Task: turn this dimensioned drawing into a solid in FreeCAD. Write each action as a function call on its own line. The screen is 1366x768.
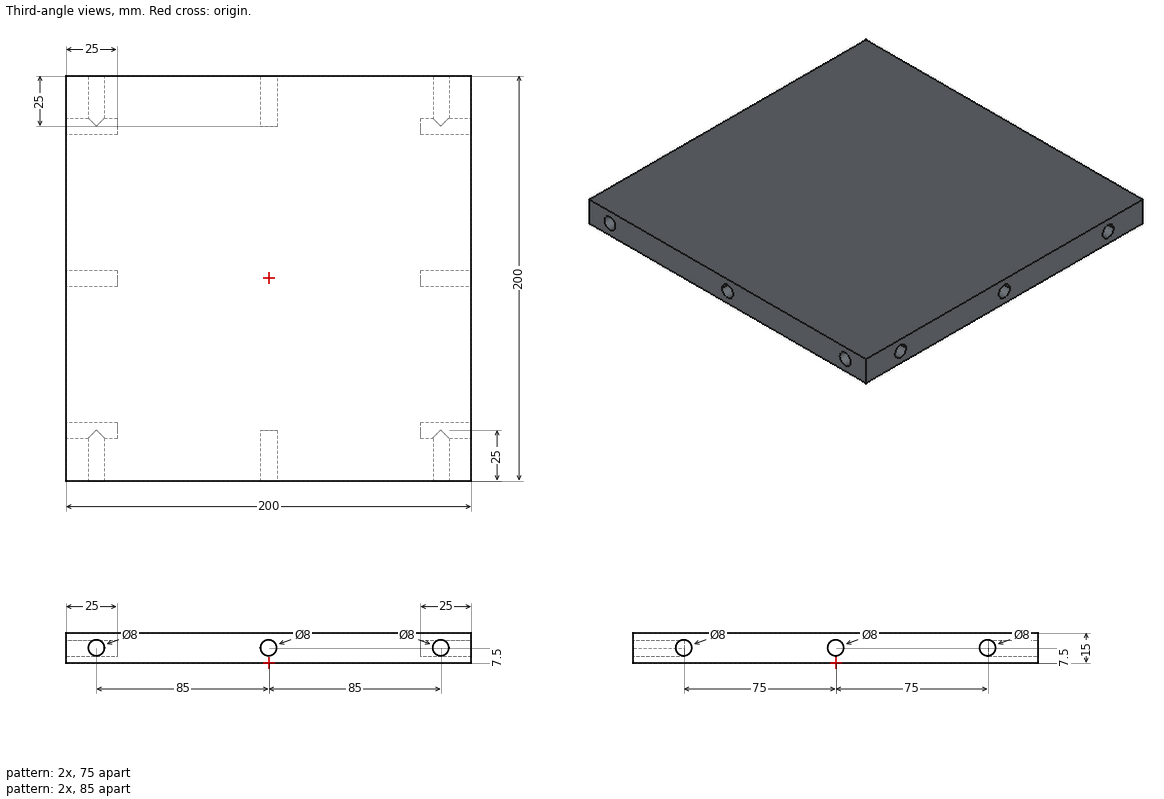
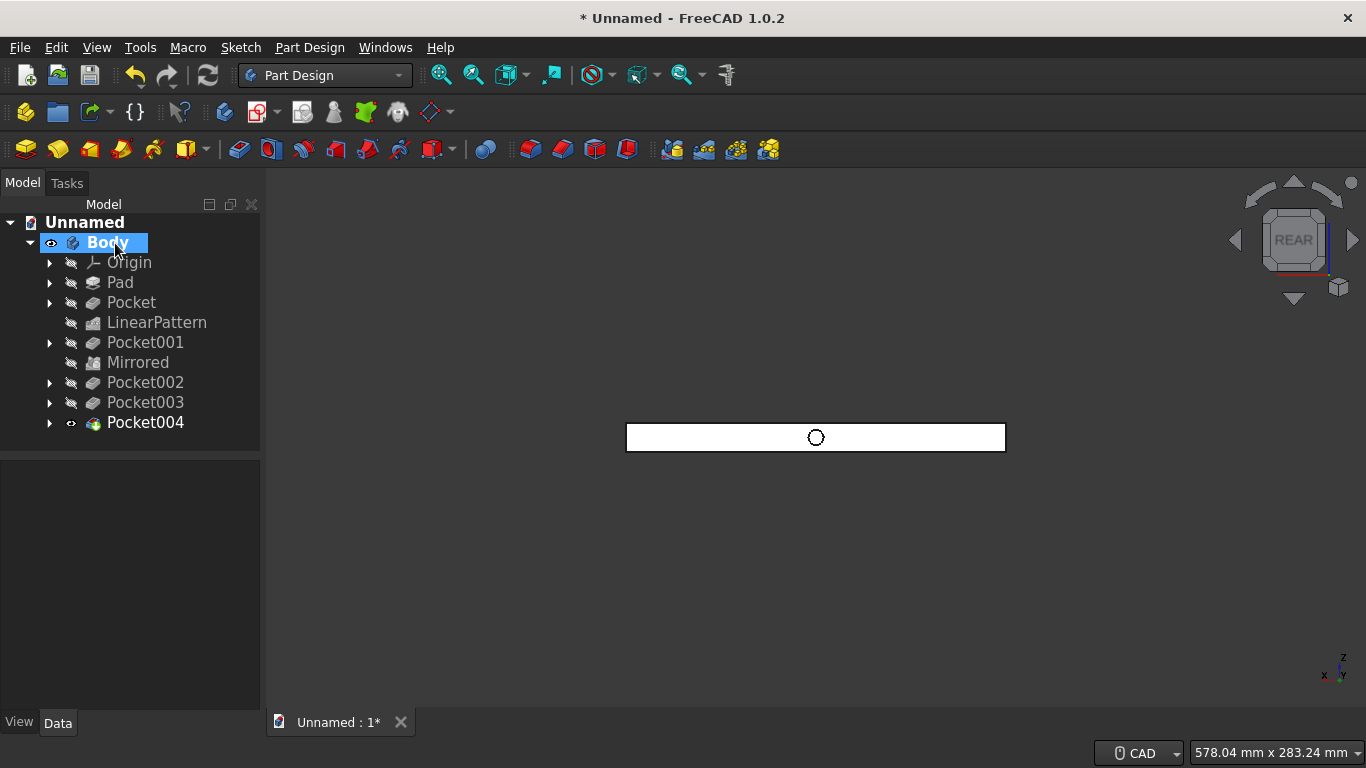
key(v)
key(f)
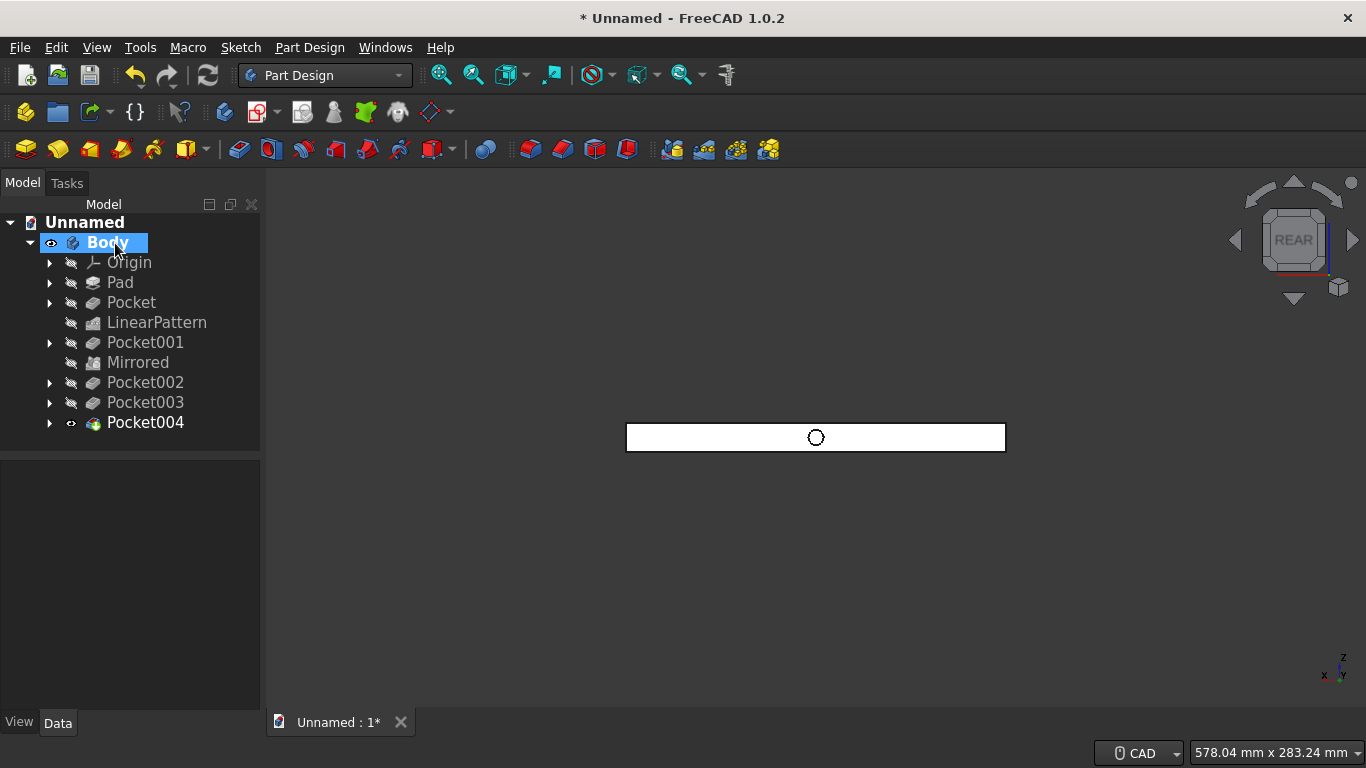
click(116, 423)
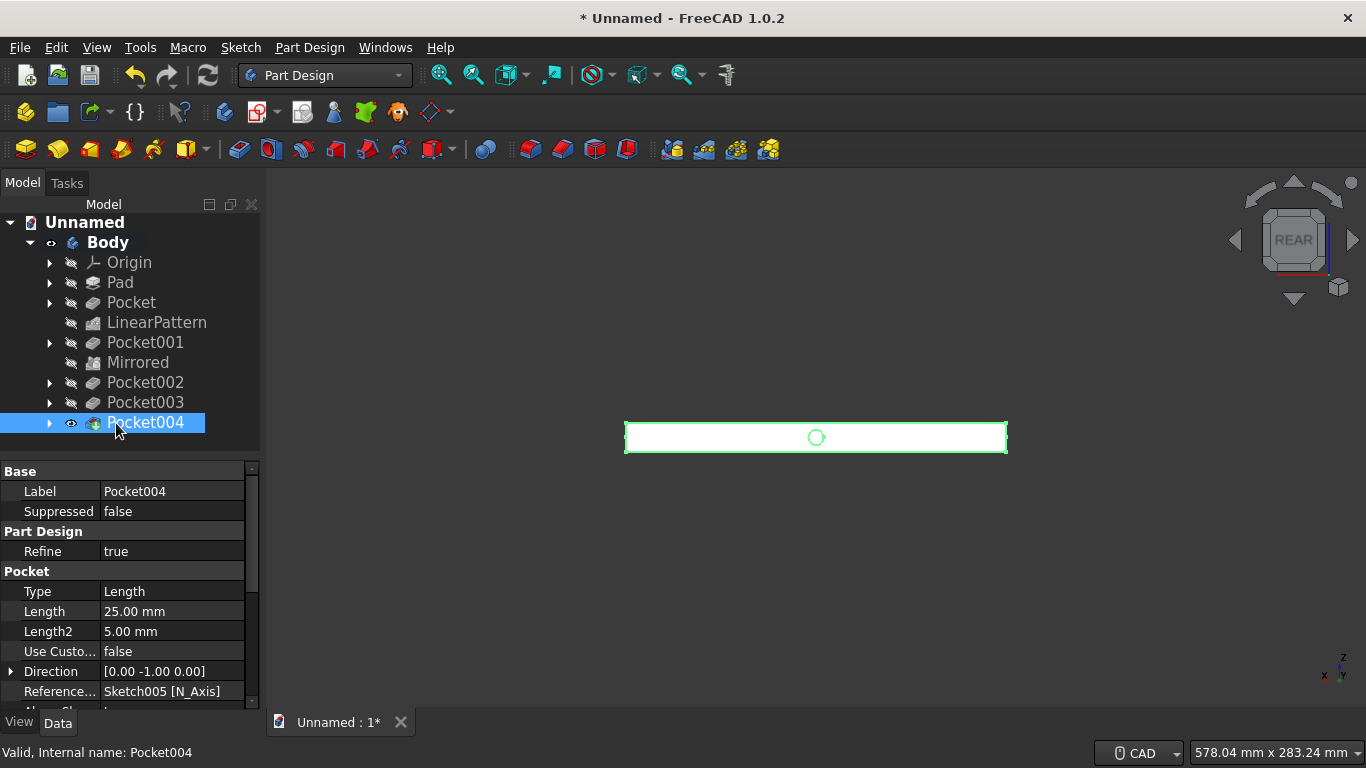
click(704, 150)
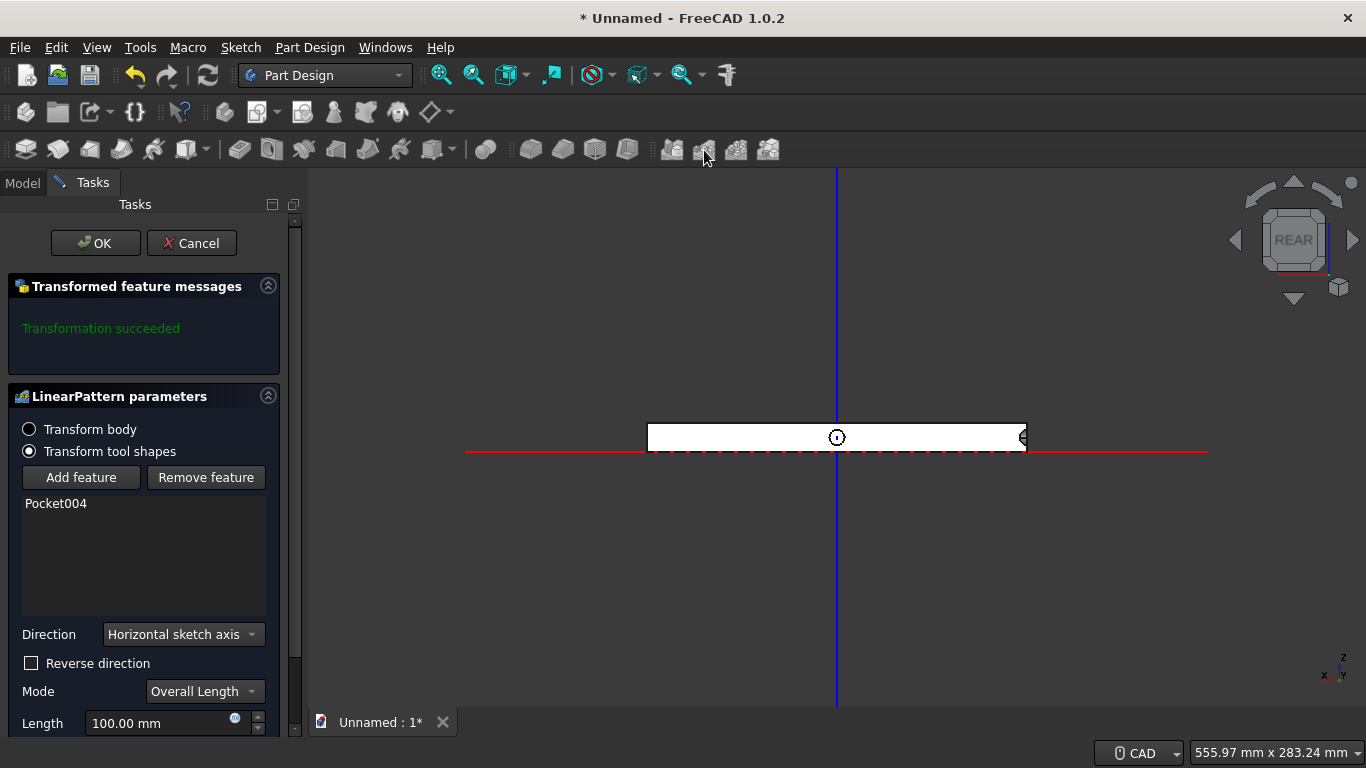
click(184, 634)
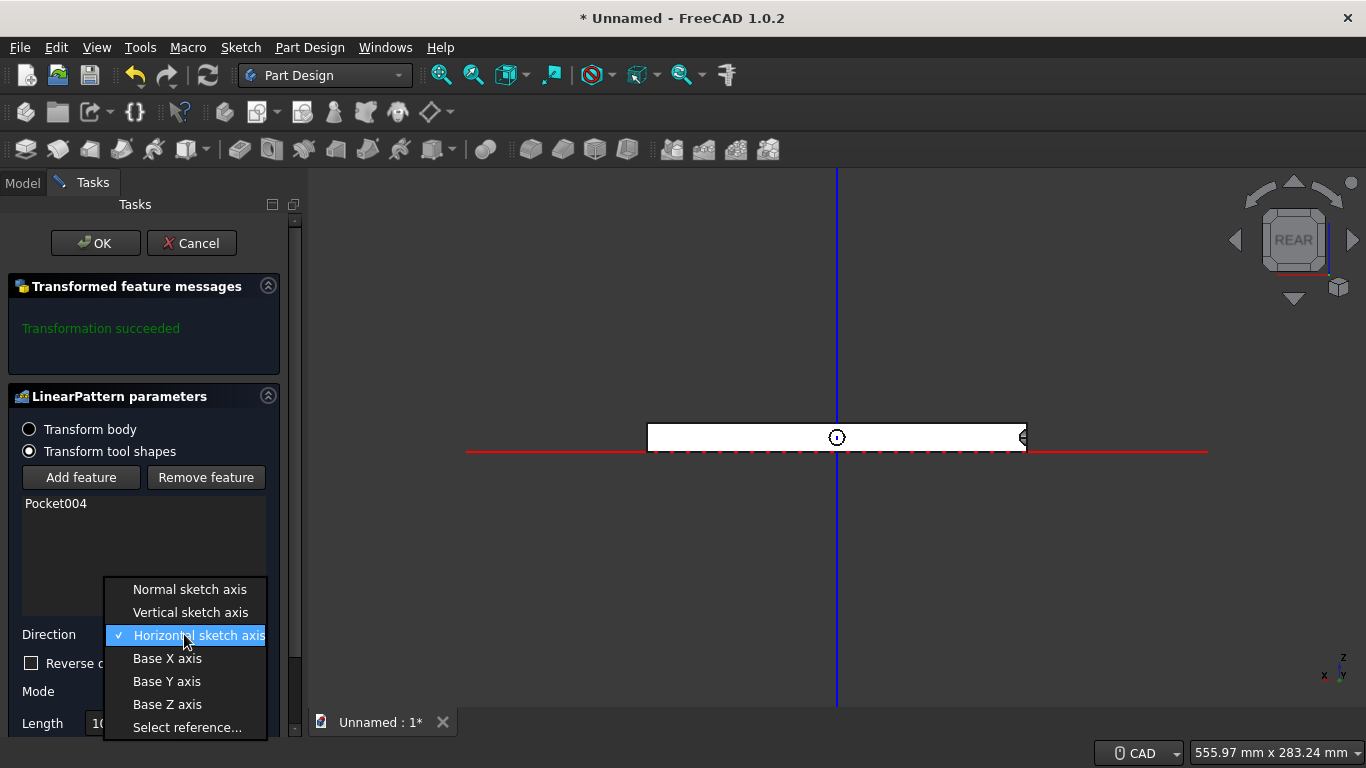
click(184, 658)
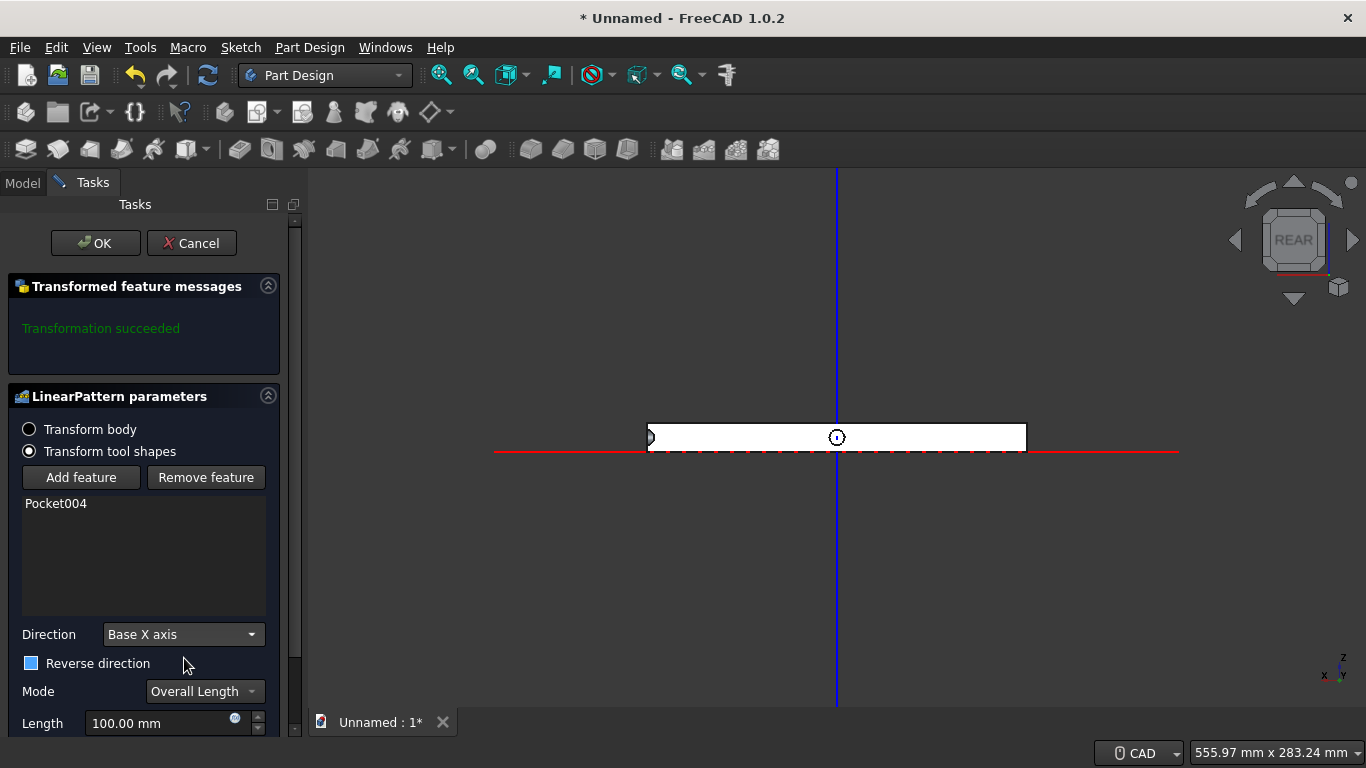
click(206, 692)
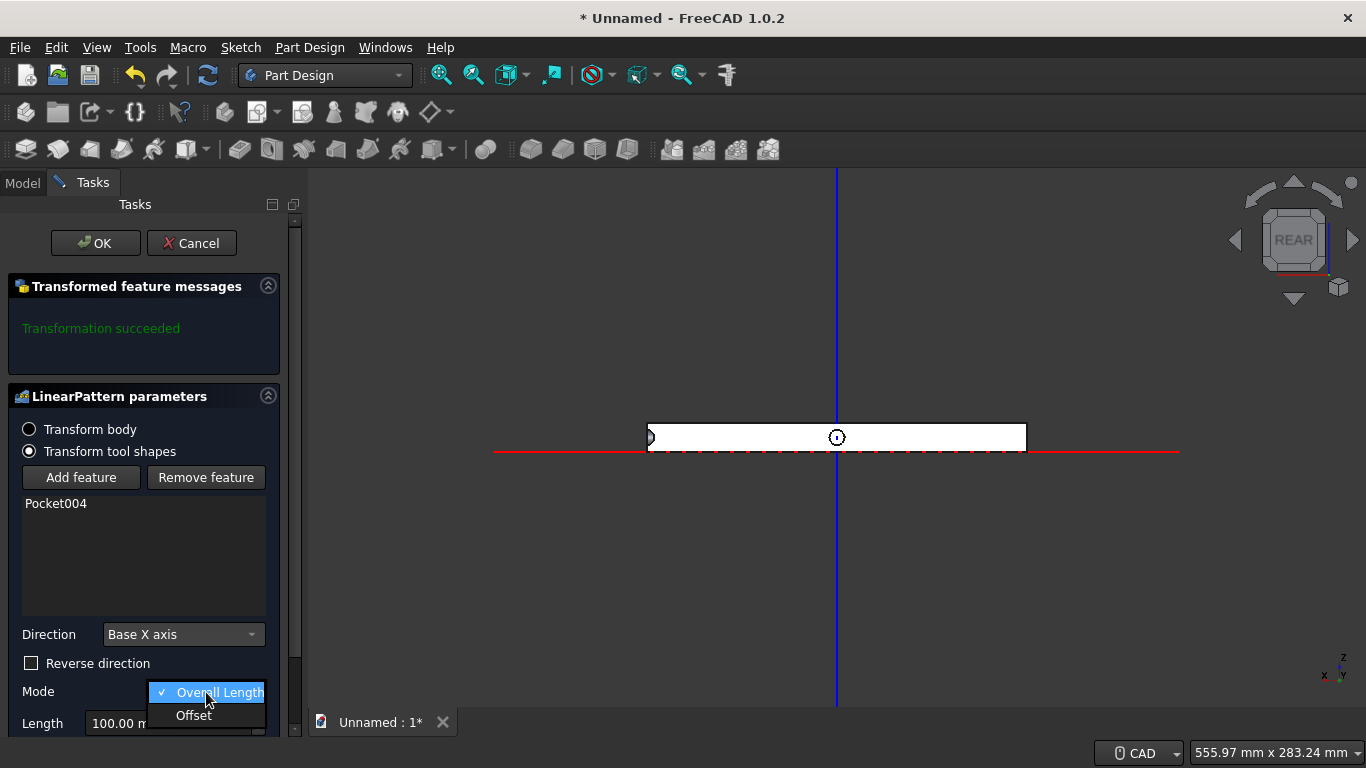
click(206, 716)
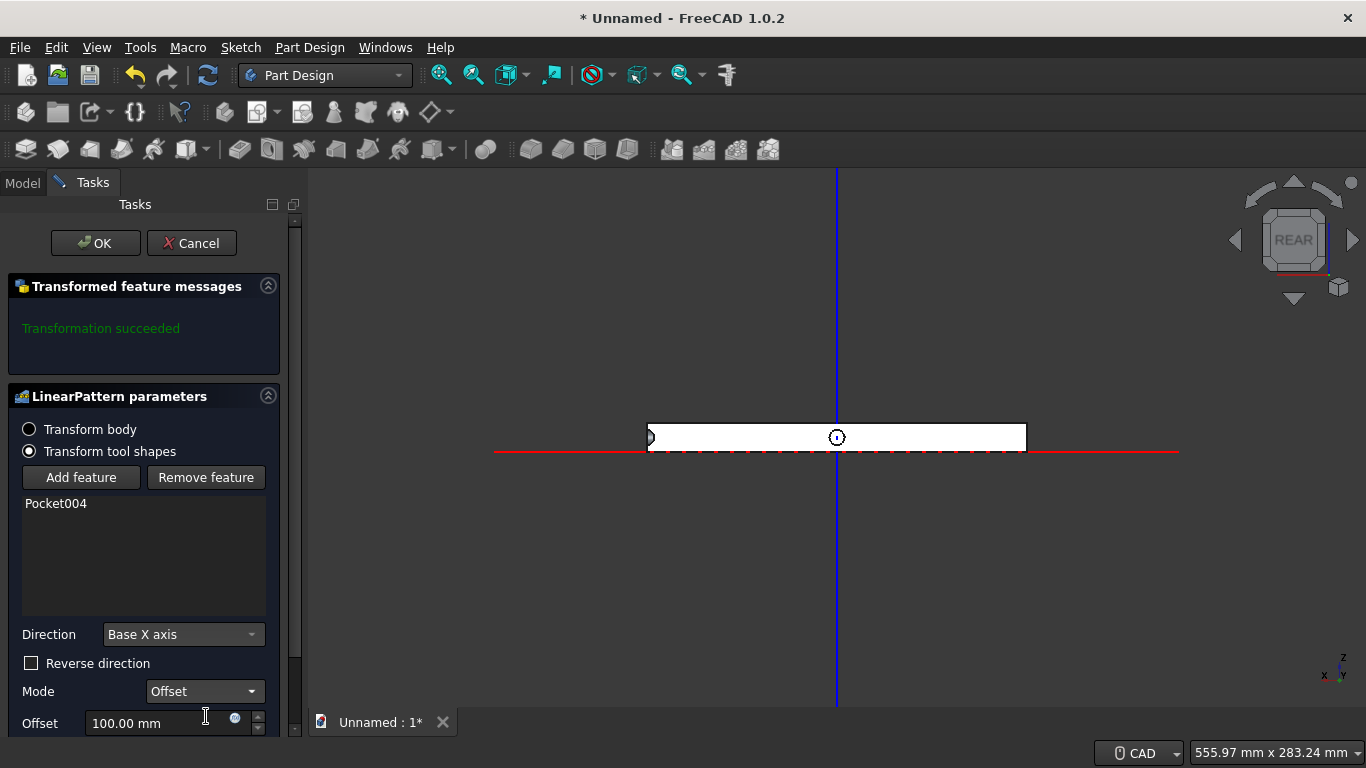
triple_click(168, 723)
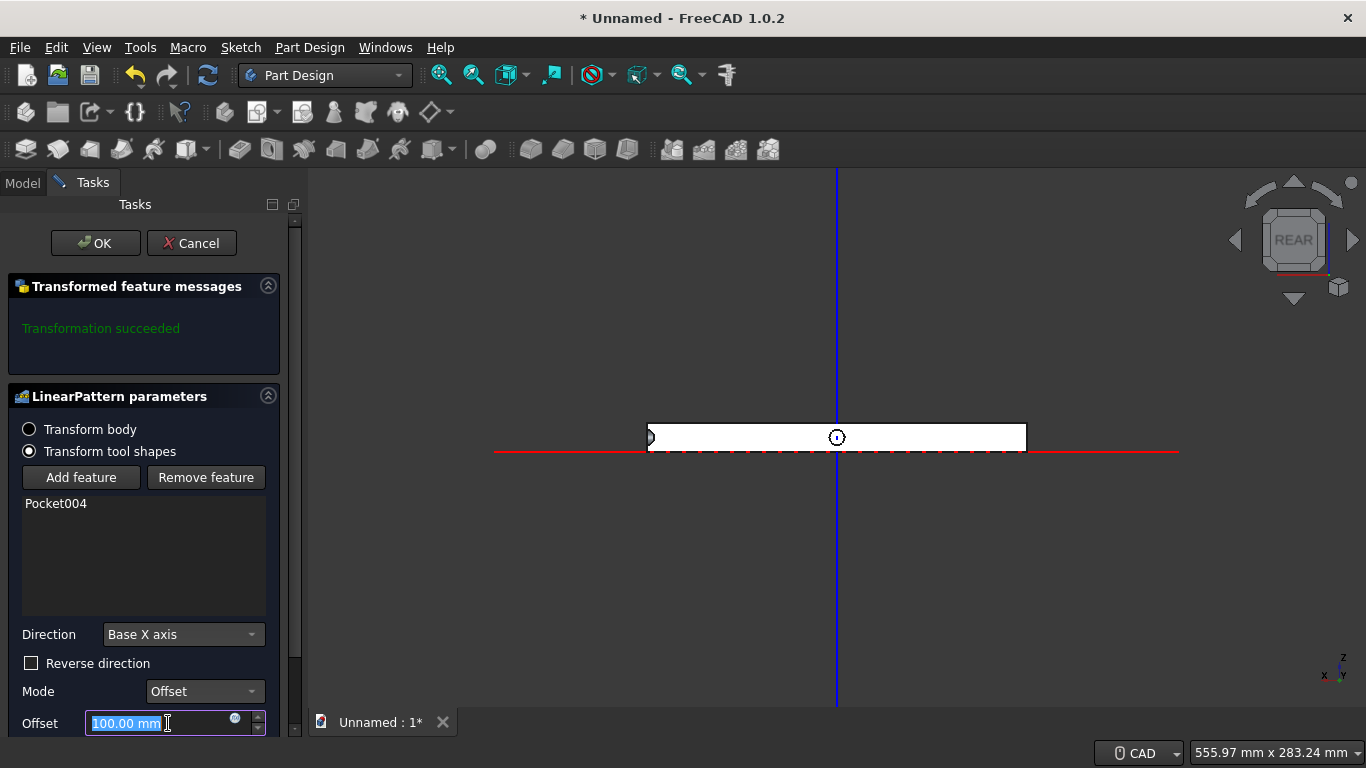
text(85)
key(Tab)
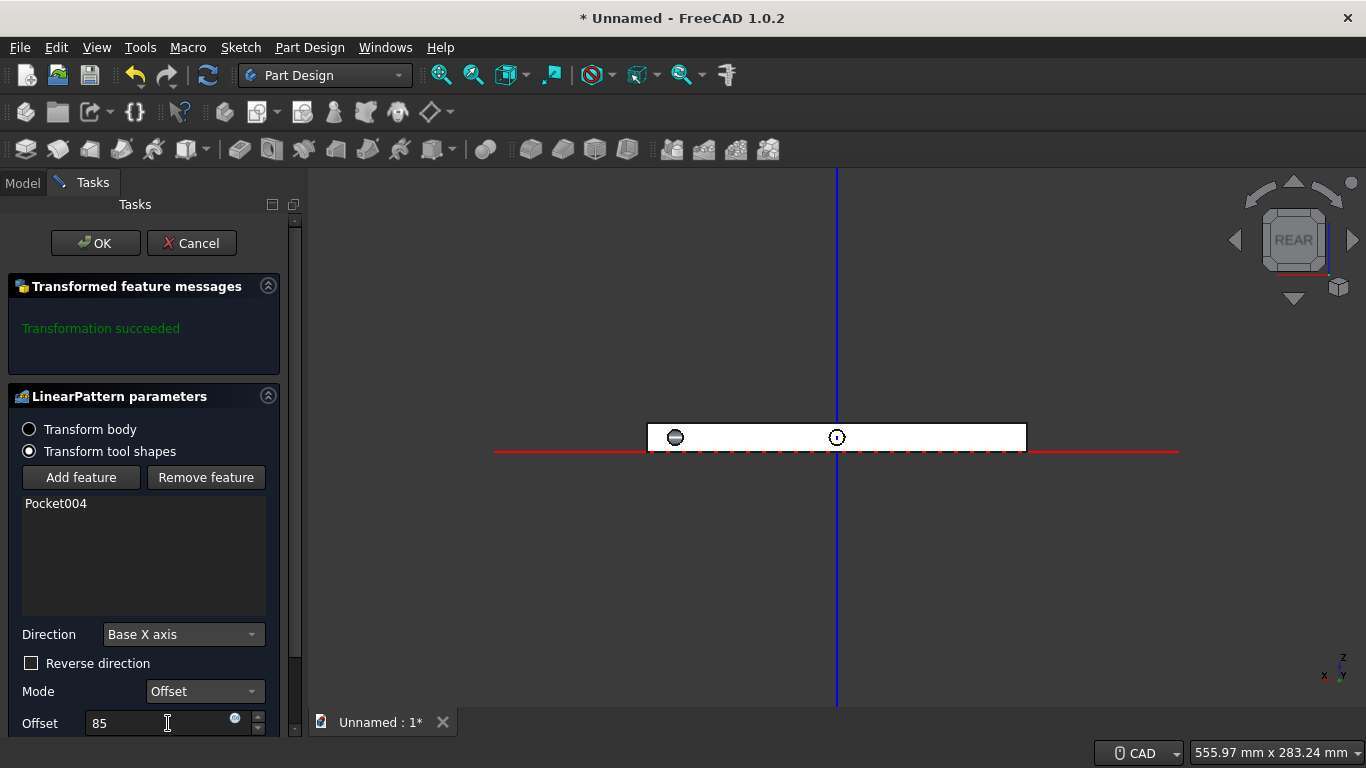
scroll(295, 475, down, 2)